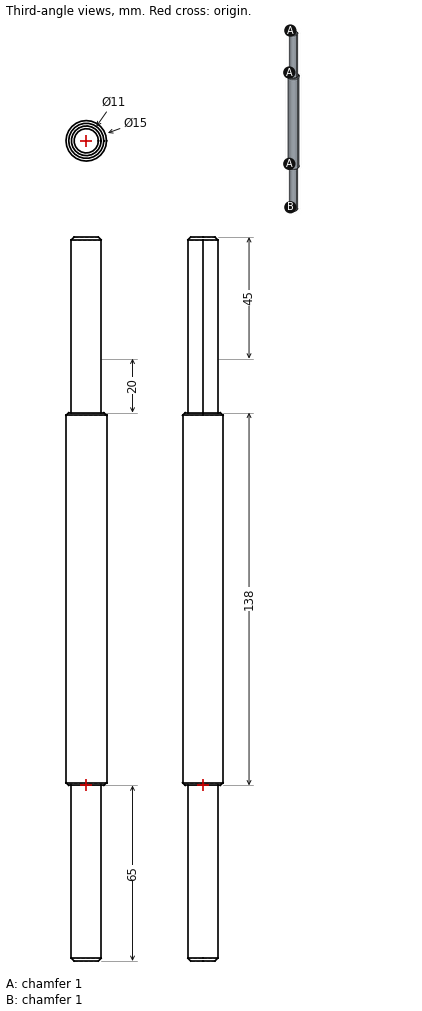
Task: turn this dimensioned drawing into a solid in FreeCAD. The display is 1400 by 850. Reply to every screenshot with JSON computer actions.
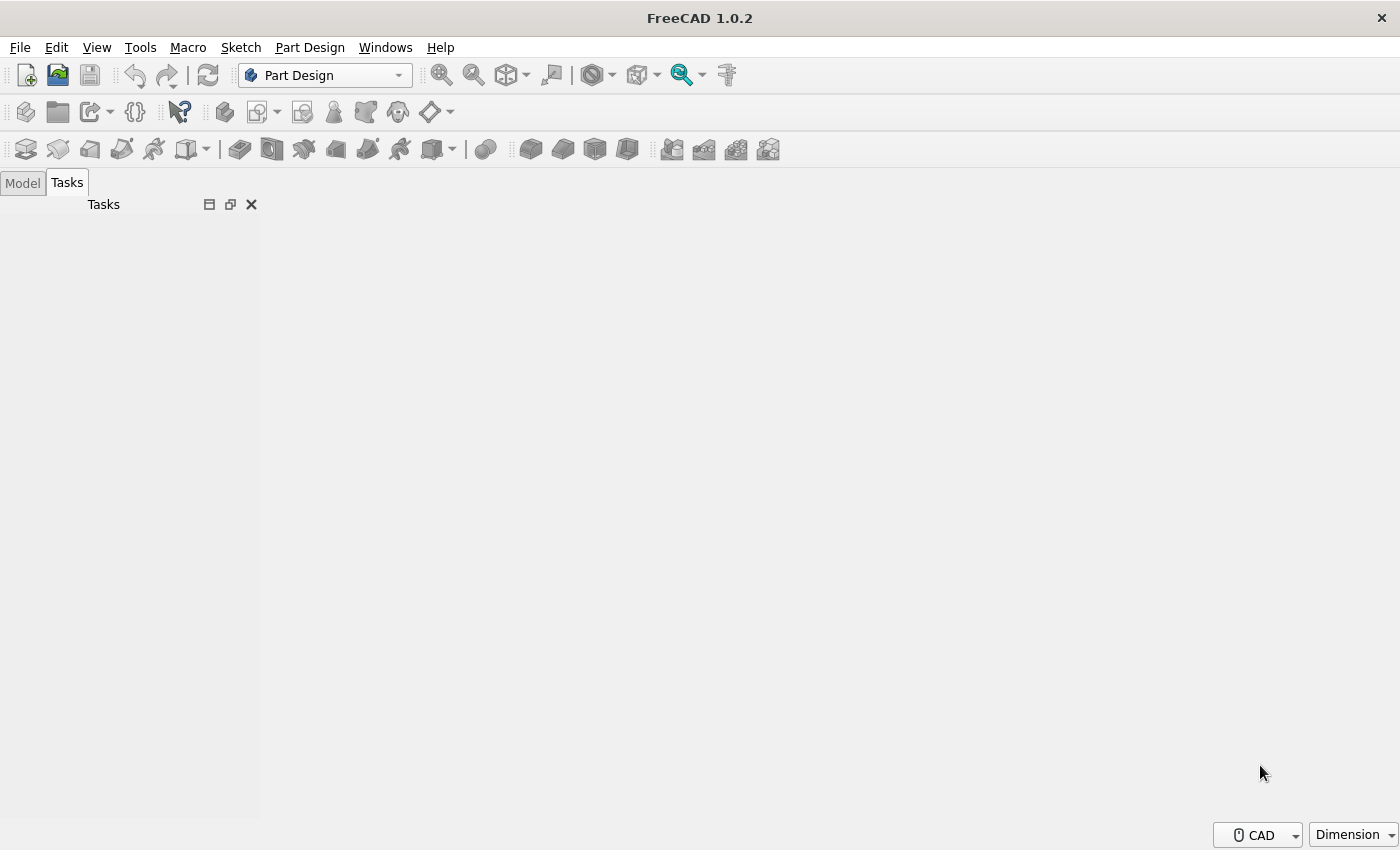
{"action": "key", "text": "ctrl+n"}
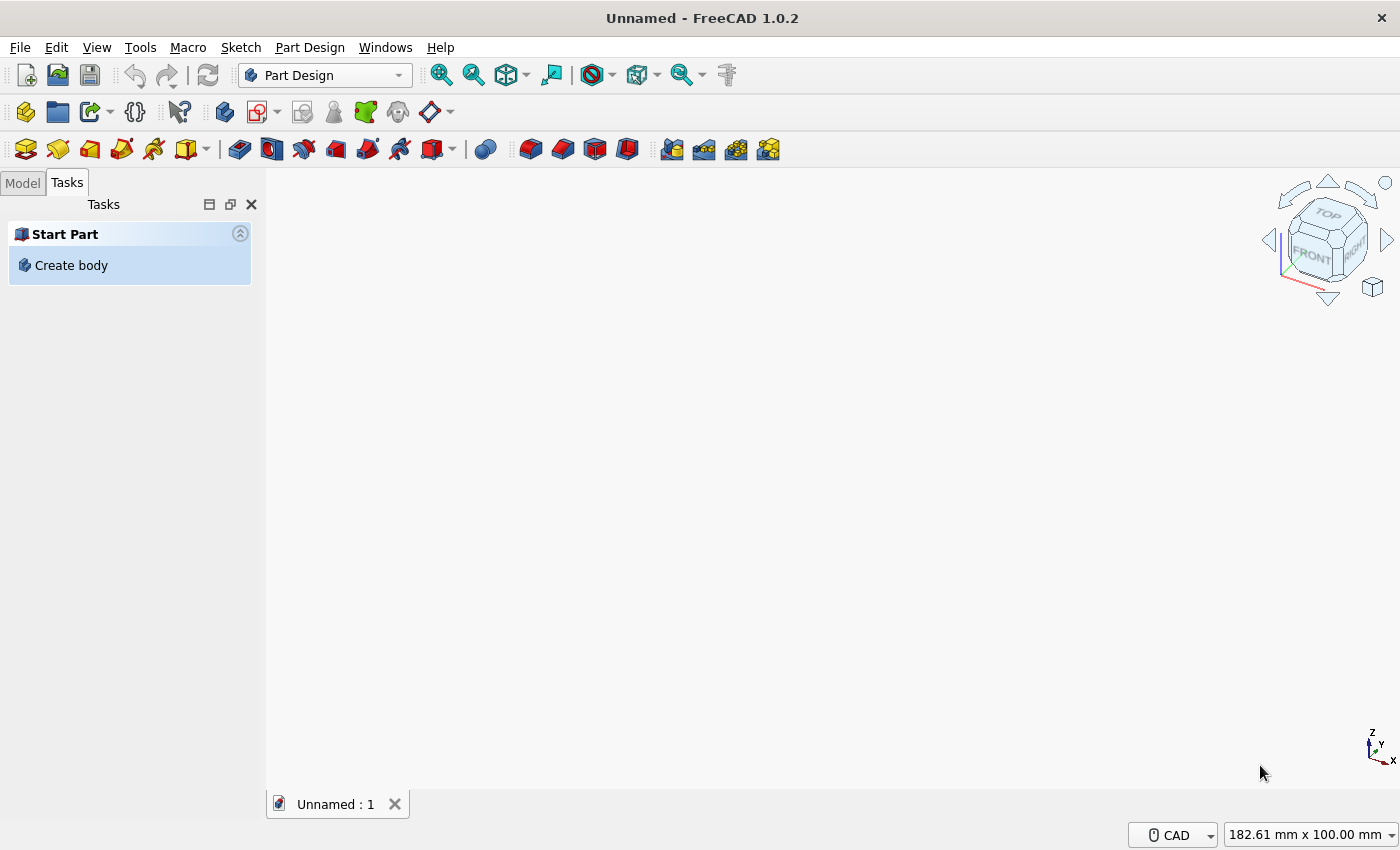
{"action": "left_click", "coordinate": [258, 112]}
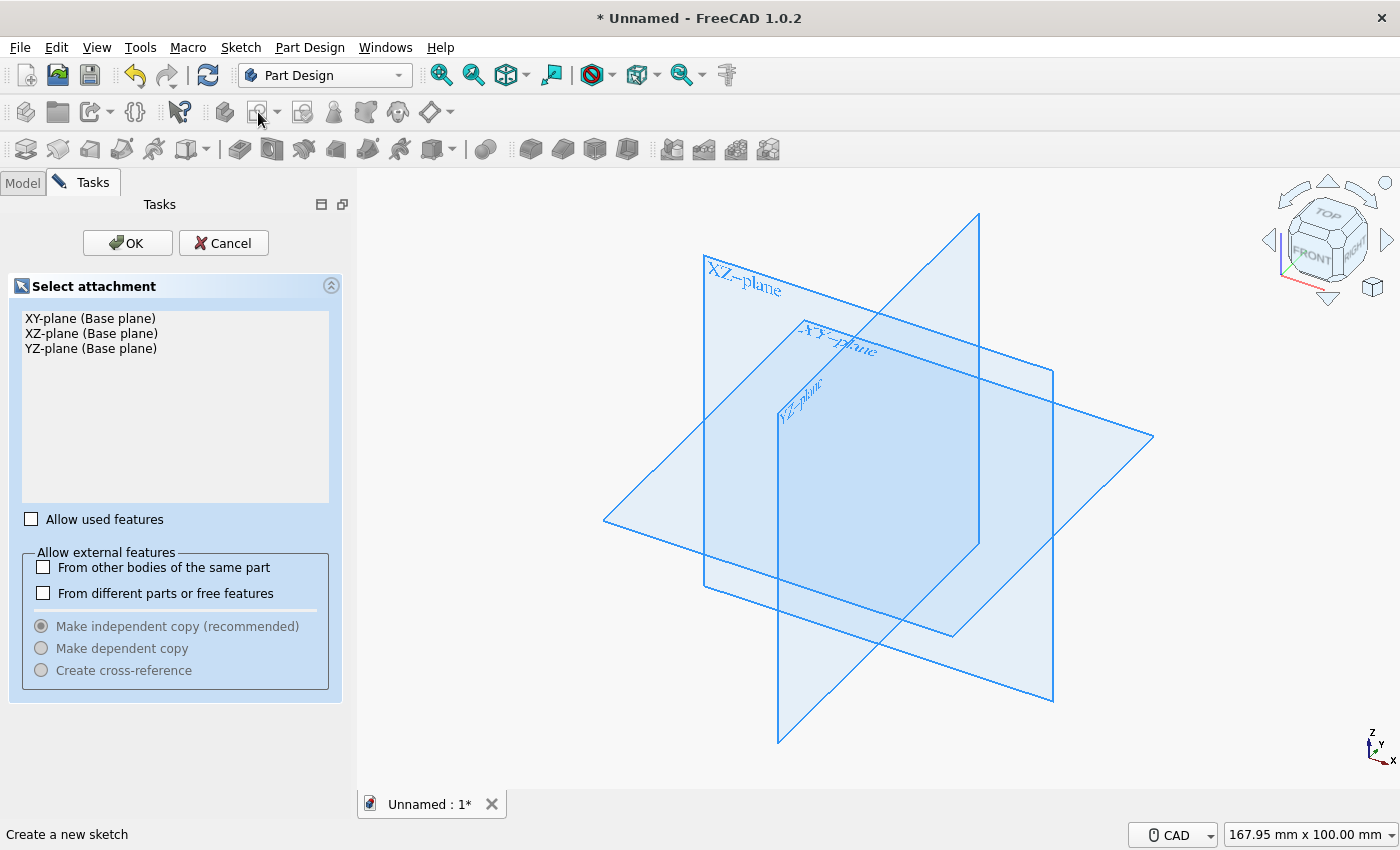
{"action": "left_click", "coordinate": [82, 318]}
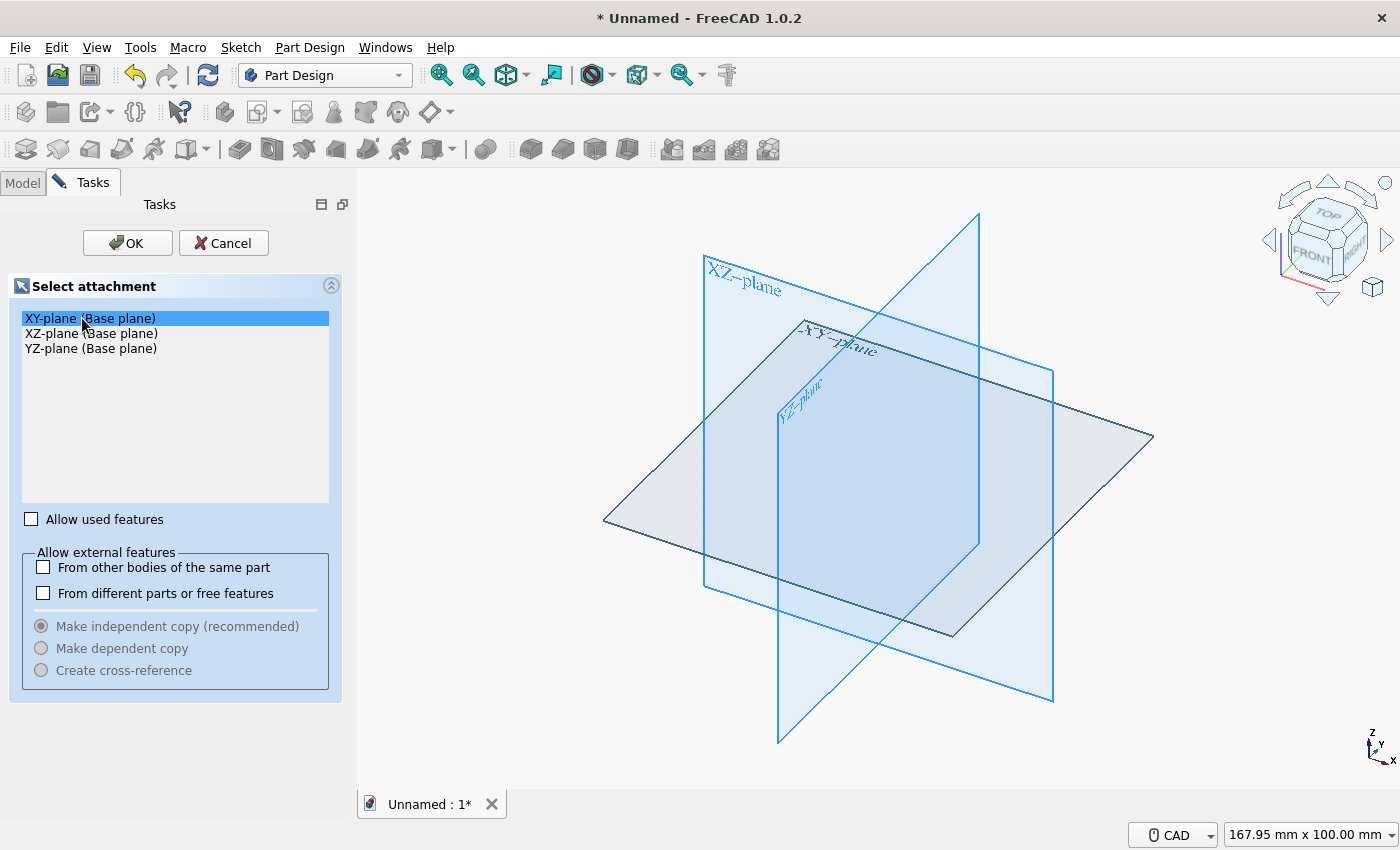
{"action": "left_click", "coordinate": [128, 243]}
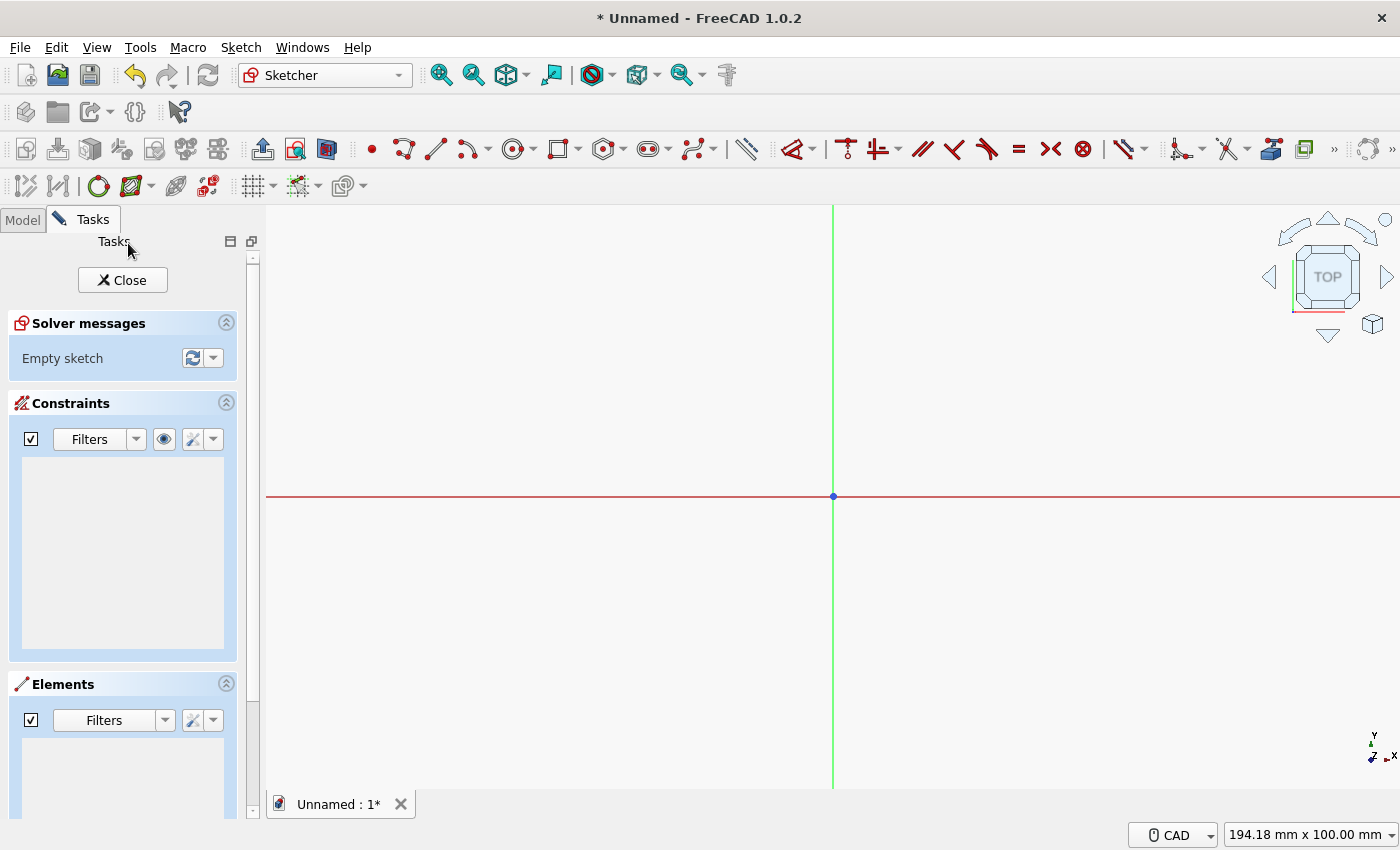
{"action": "scroll", "coordinate": [855, 497], "scroll_direction": "up", "scroll_amount": 7}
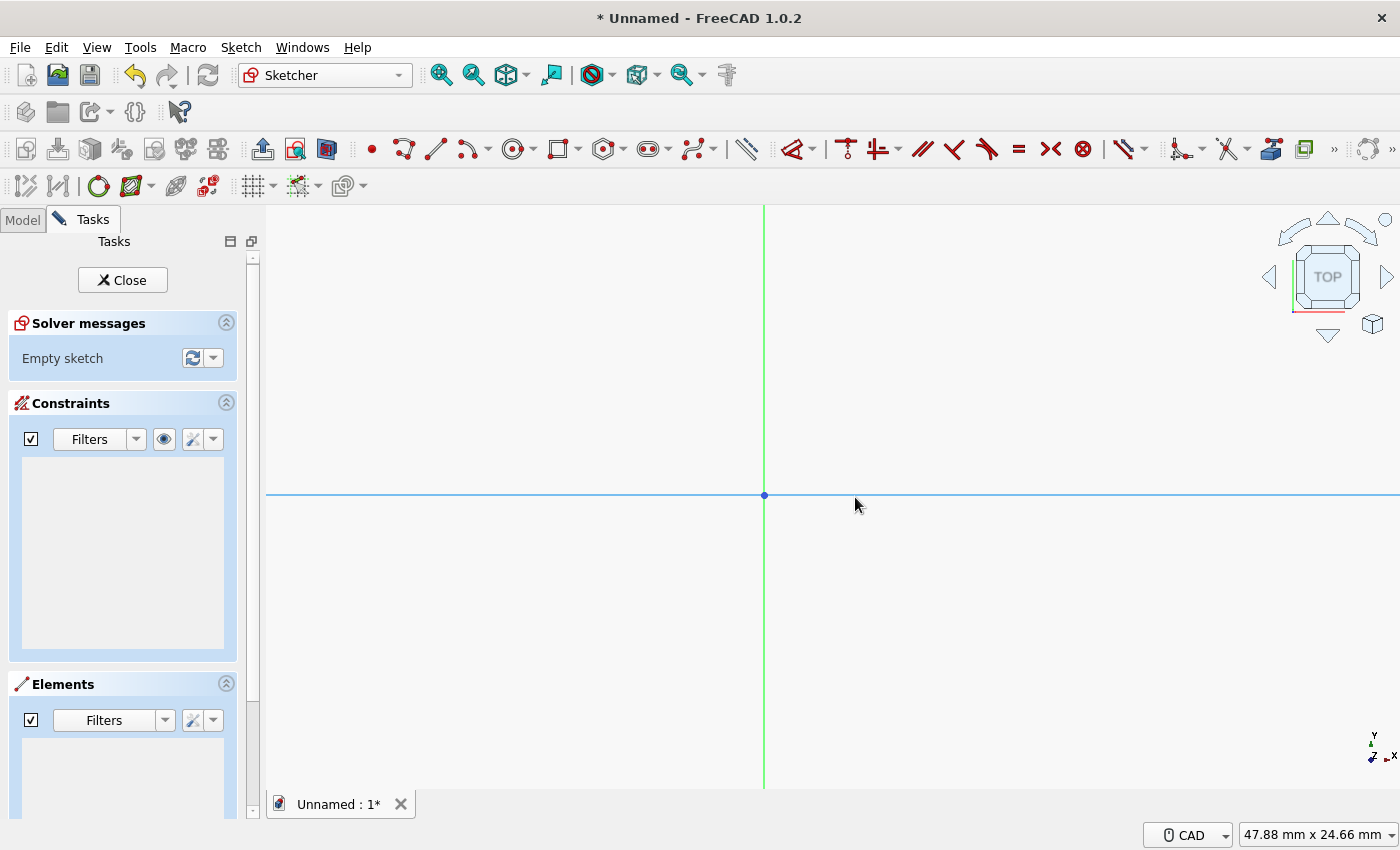
{"action": "key", "text": "g c"}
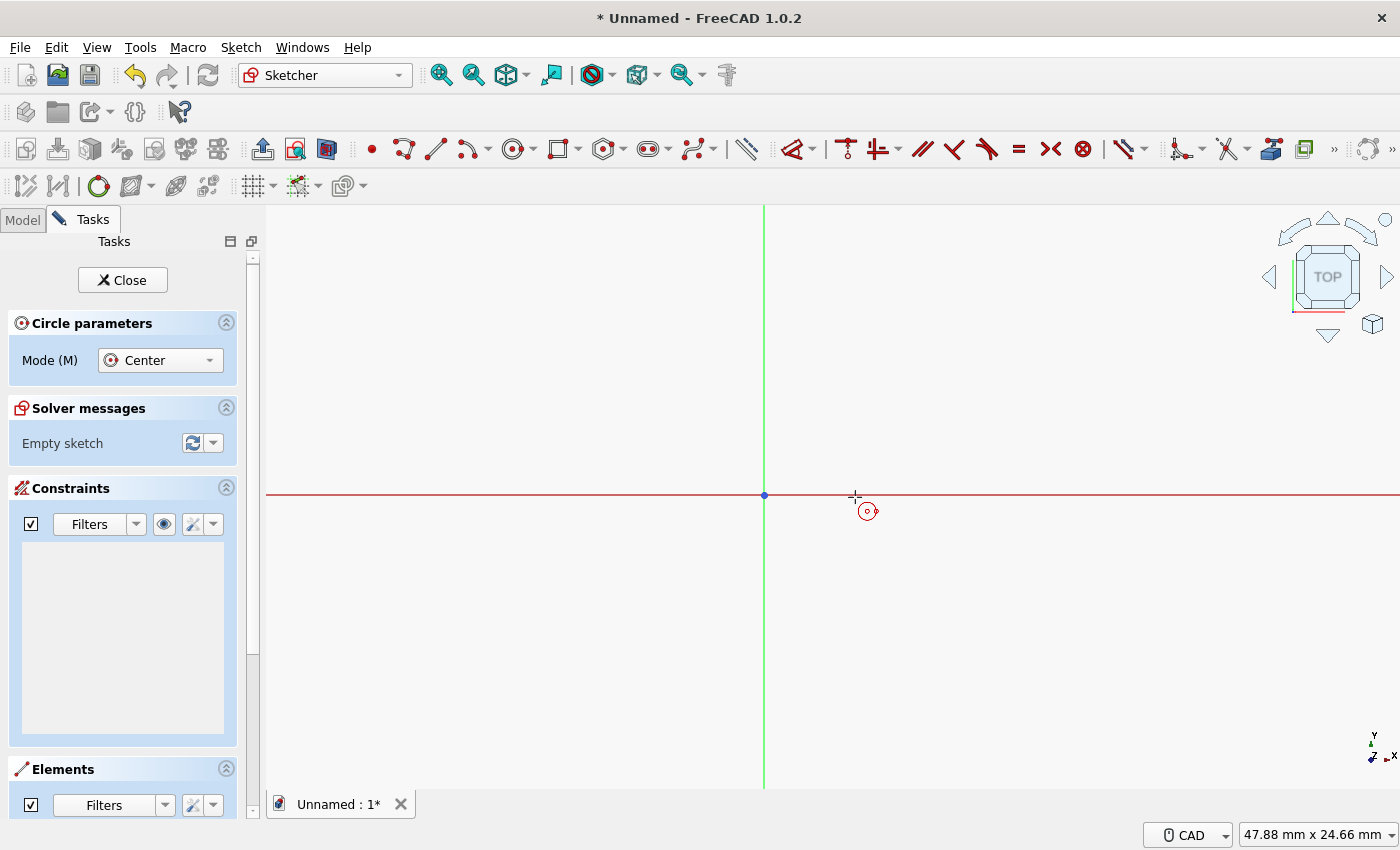
{"action": "left_click", "coordinate": [764, 495]}
{"action": "mouse_move", "coordinate": [890, 370]}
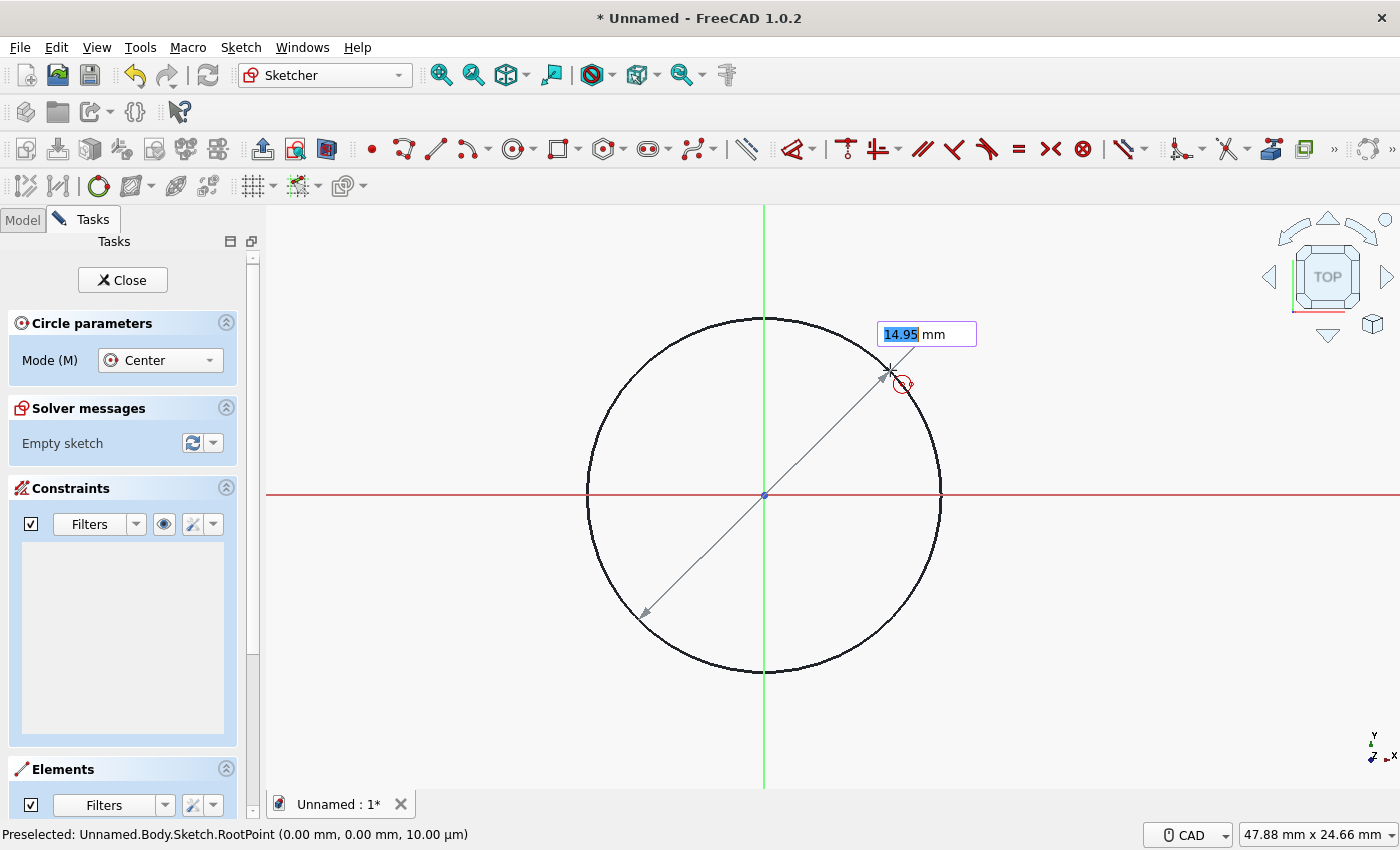
{"action": "type", "text": "15"}
{"action": "key", "text": "Return"}
{"action": "key", "text": "Escape"}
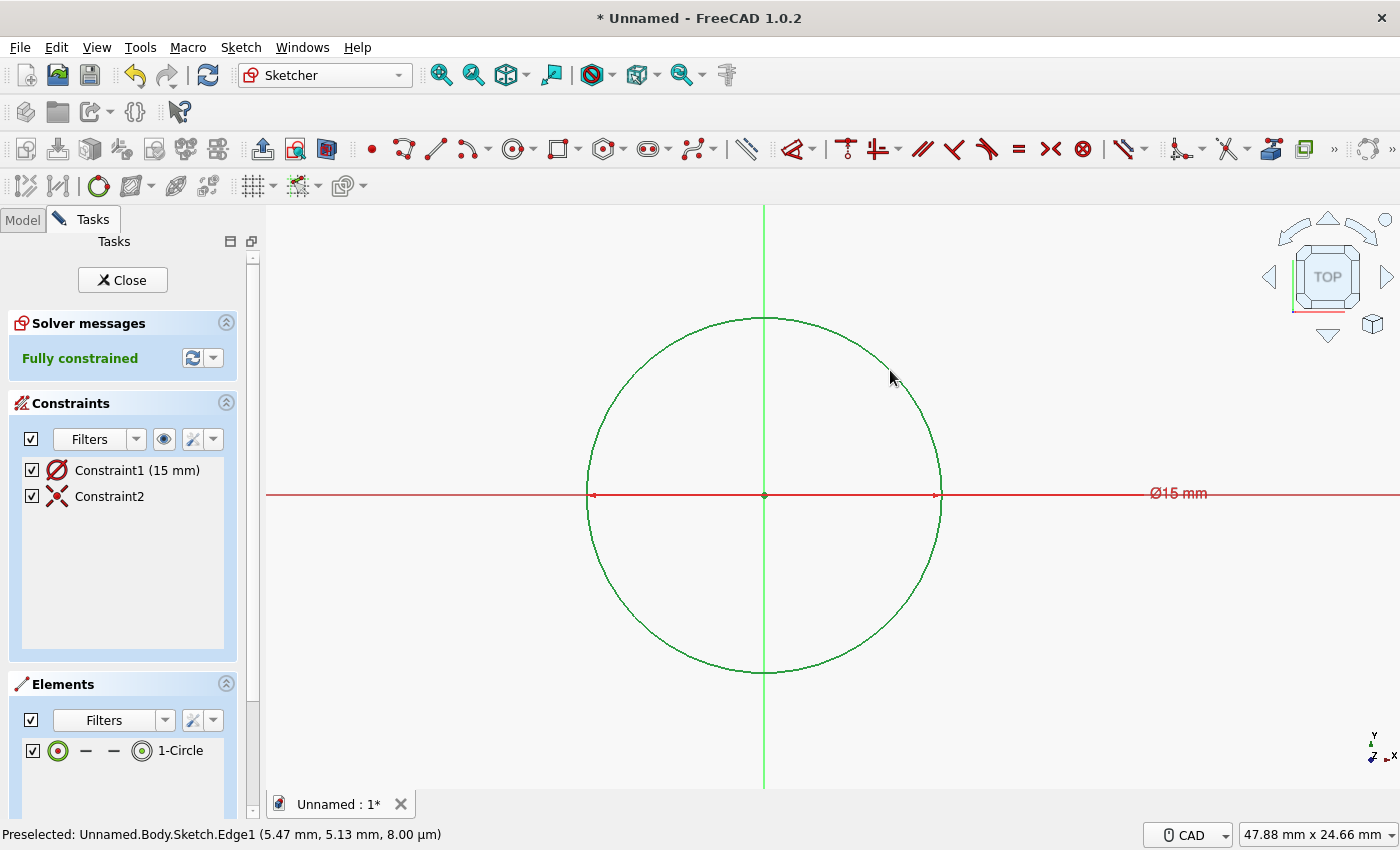
{"action": "left_click", "coordinate": [123, 280]}